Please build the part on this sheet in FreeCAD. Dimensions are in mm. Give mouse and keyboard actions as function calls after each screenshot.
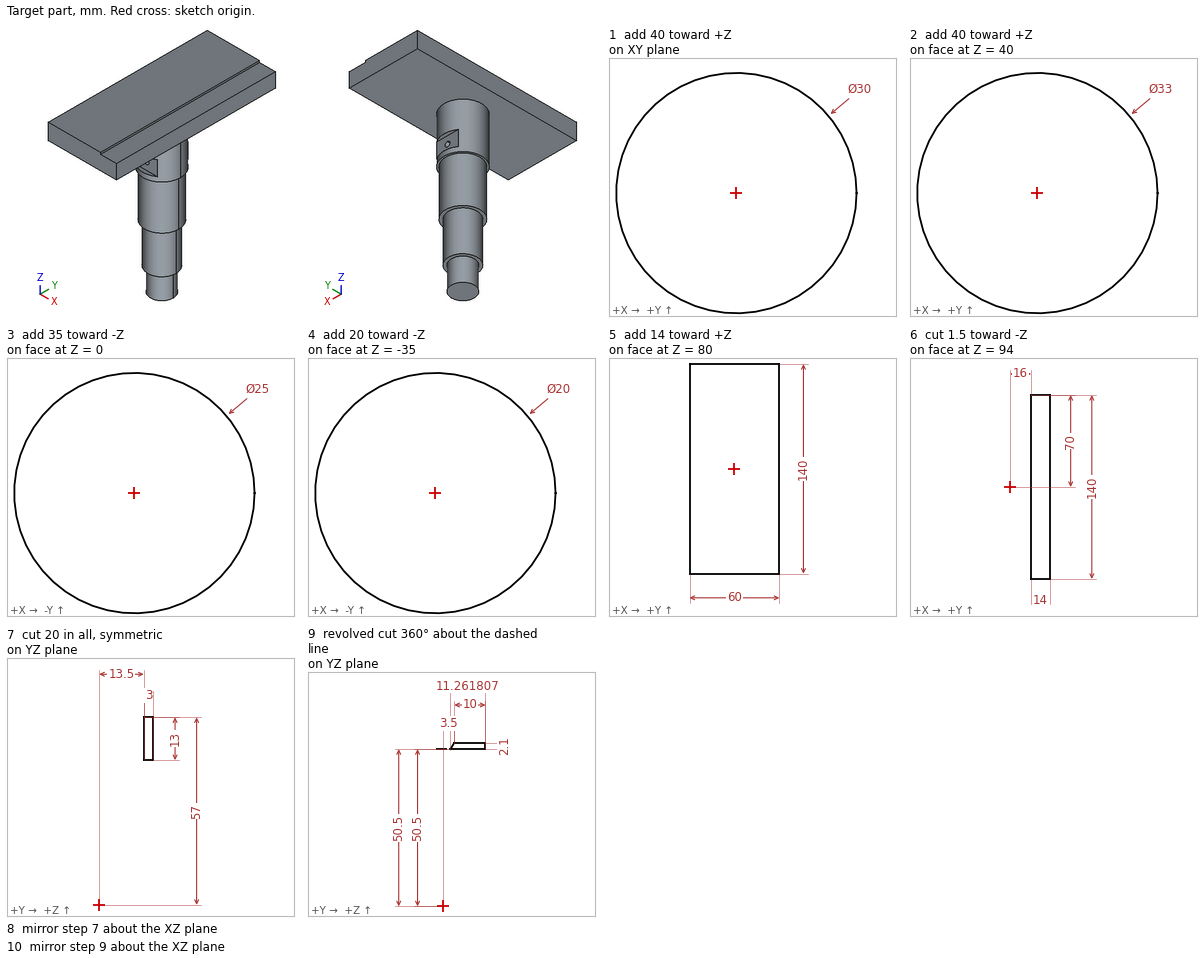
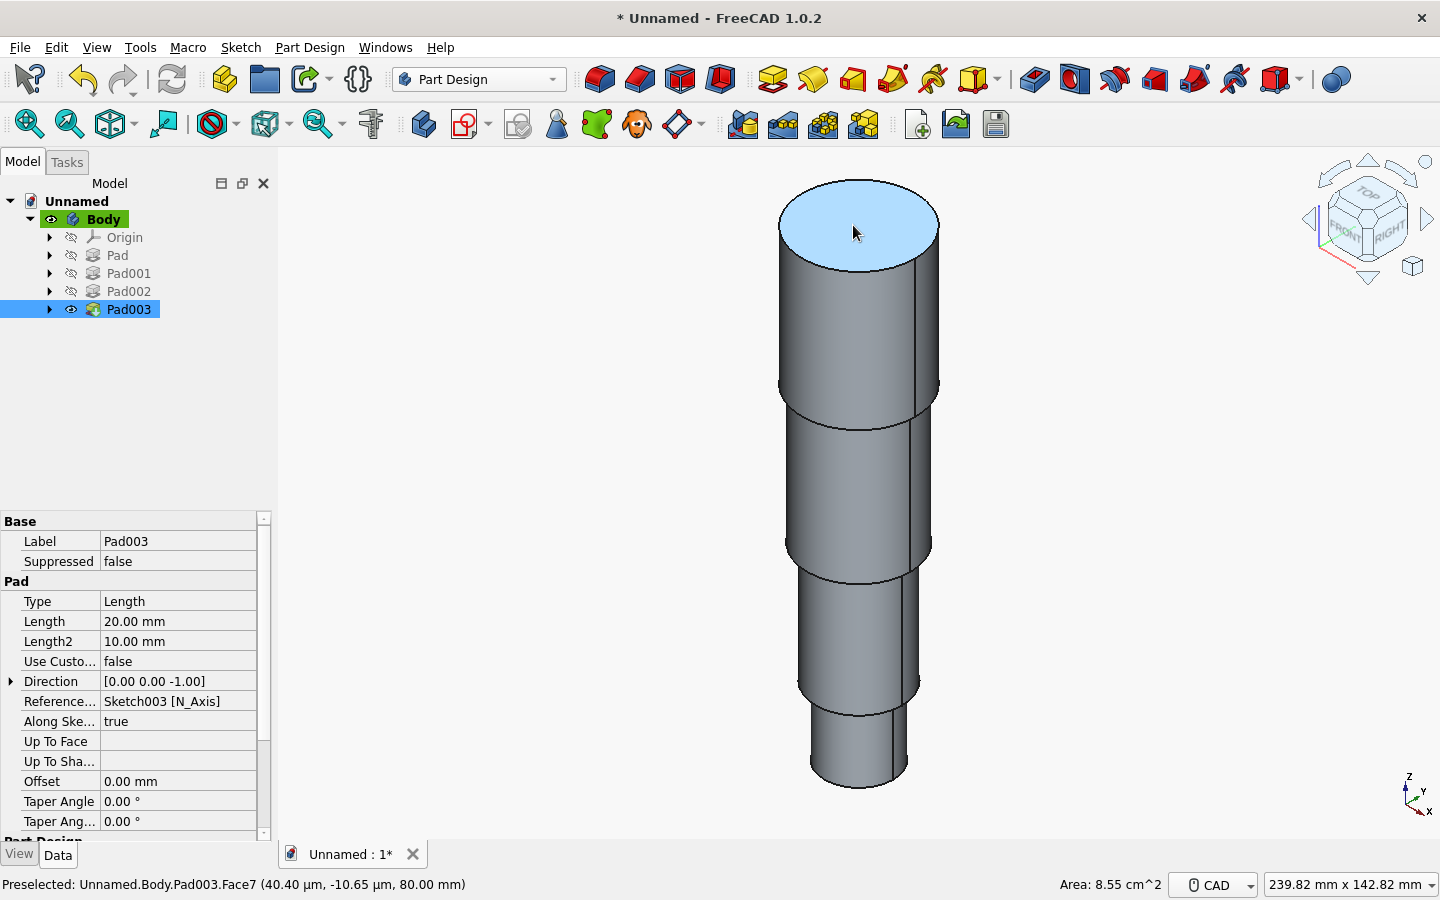
click(464, 124)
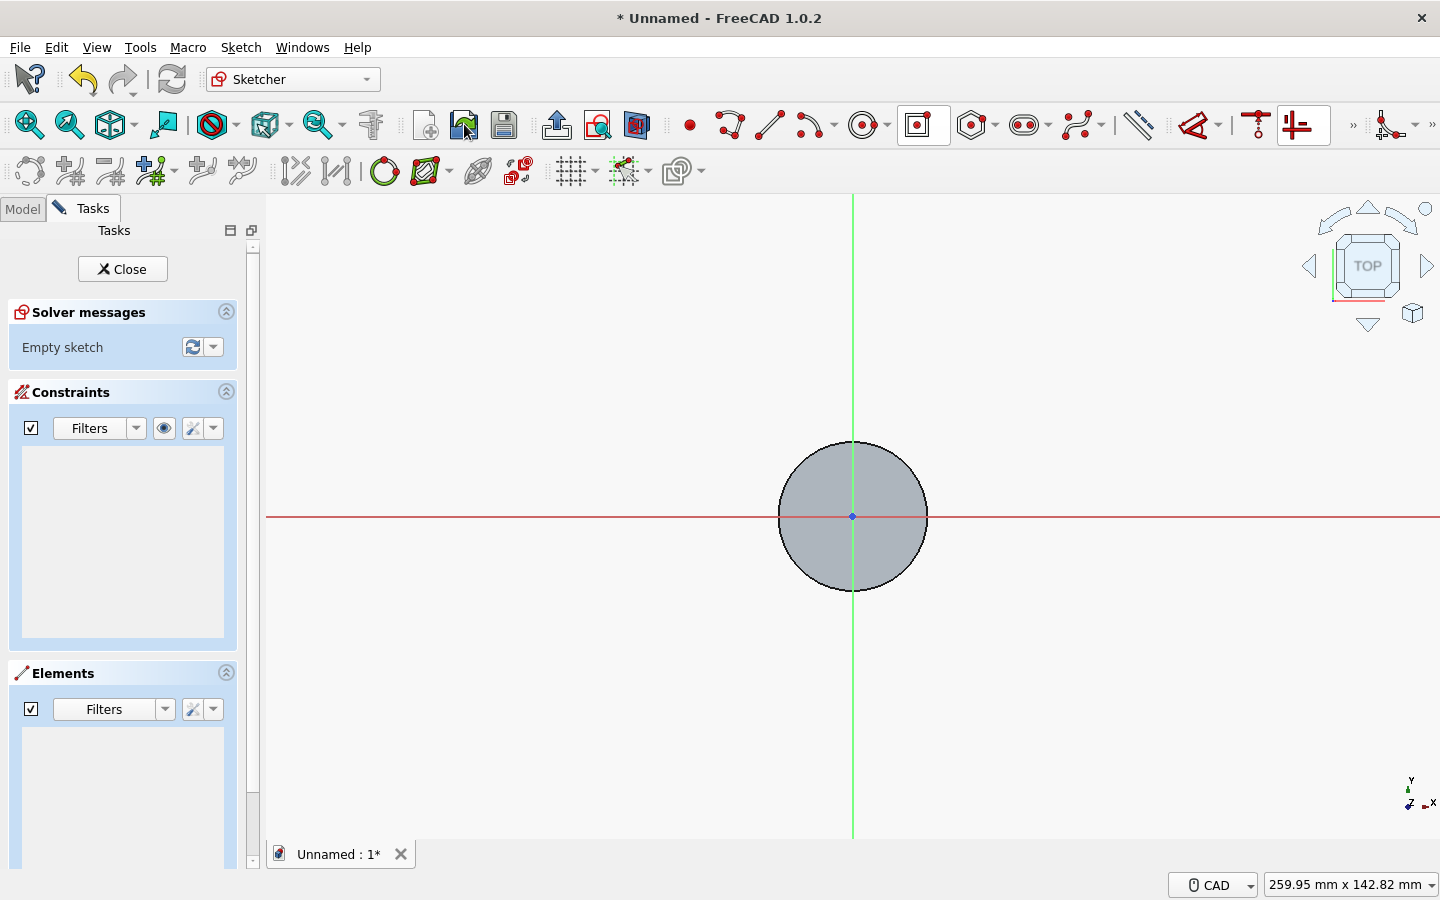
scroll(645, 516, down, 2)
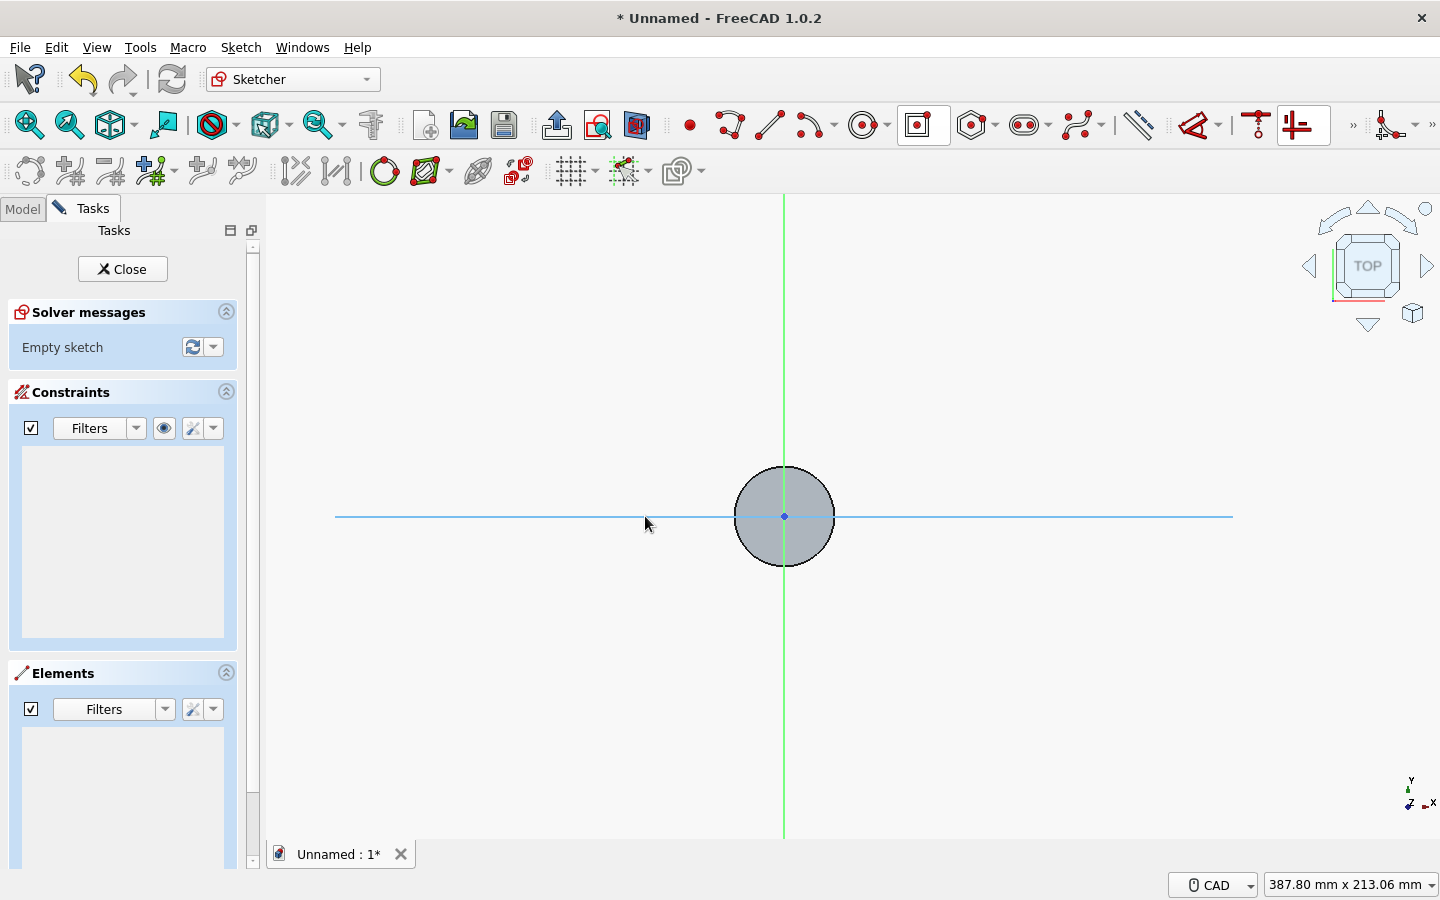
click(918, 126)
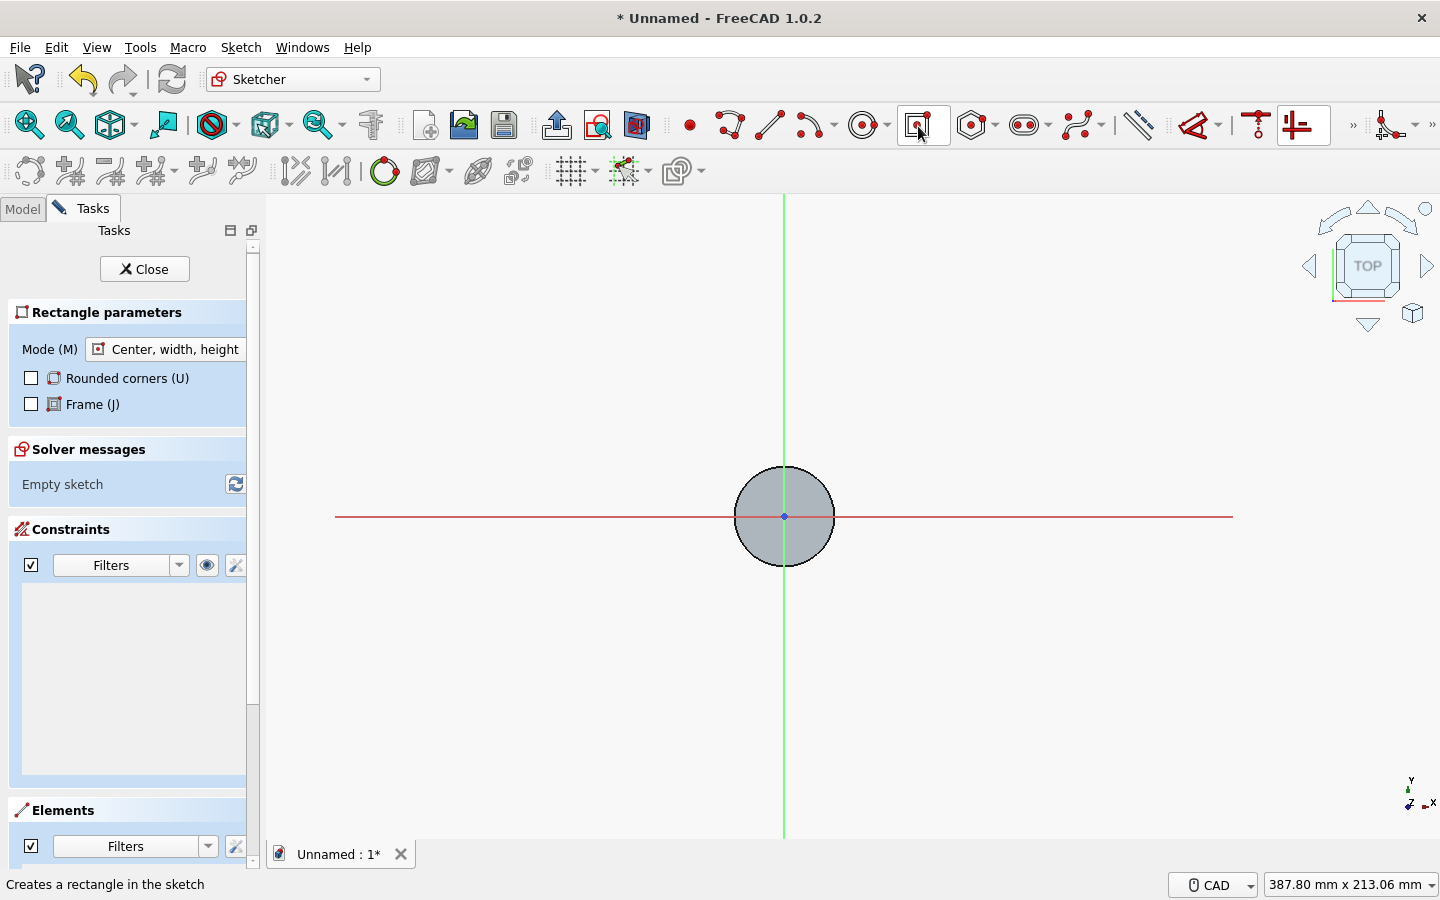
click(784, 516)
move(875, 305)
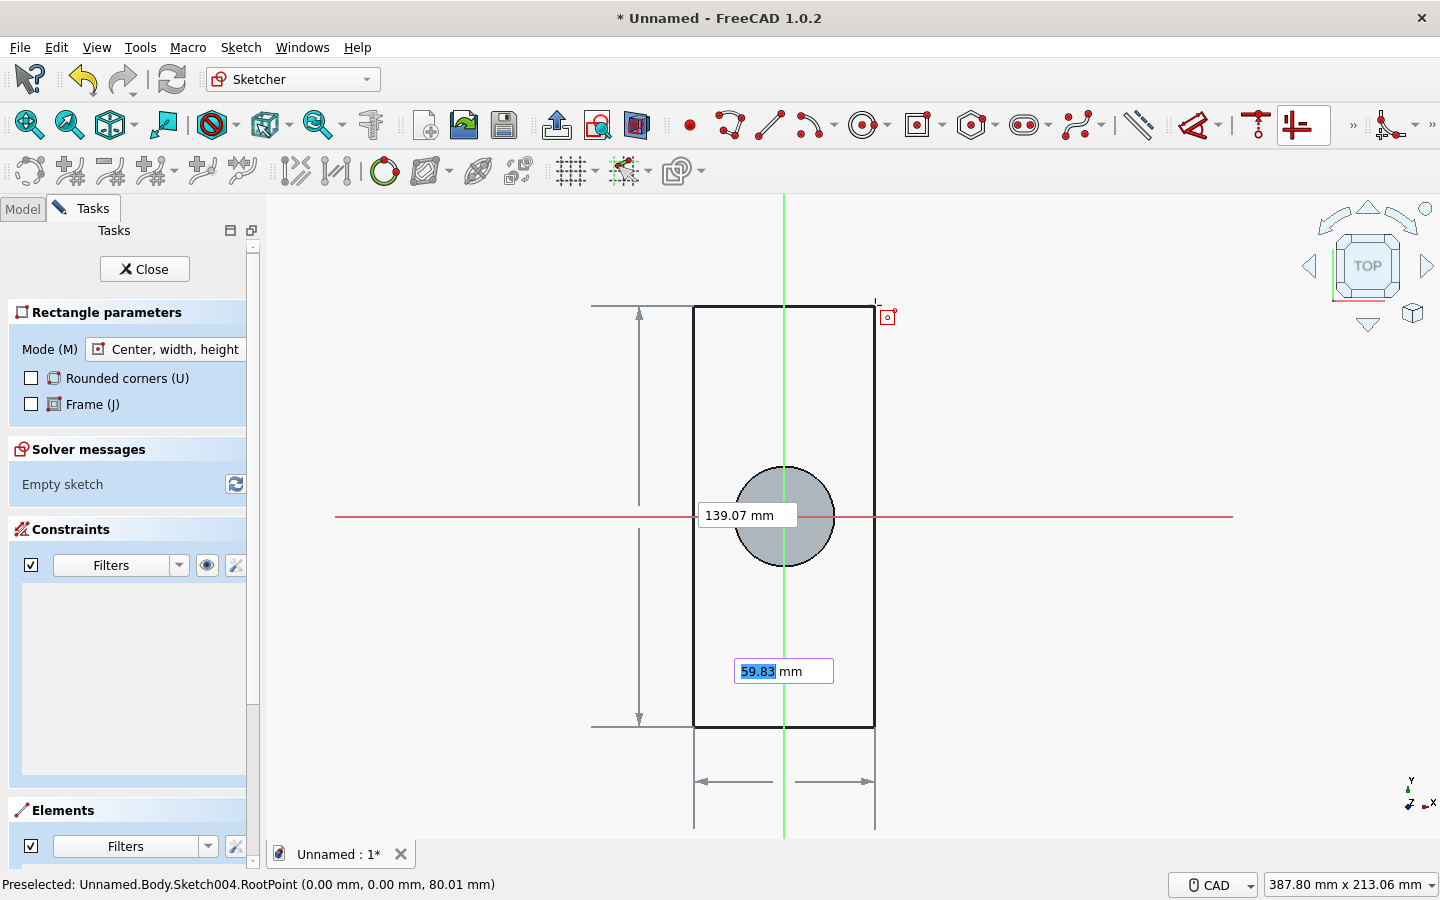
text(60)
key(Tab)
text(140)
key(Return)
key(Escape)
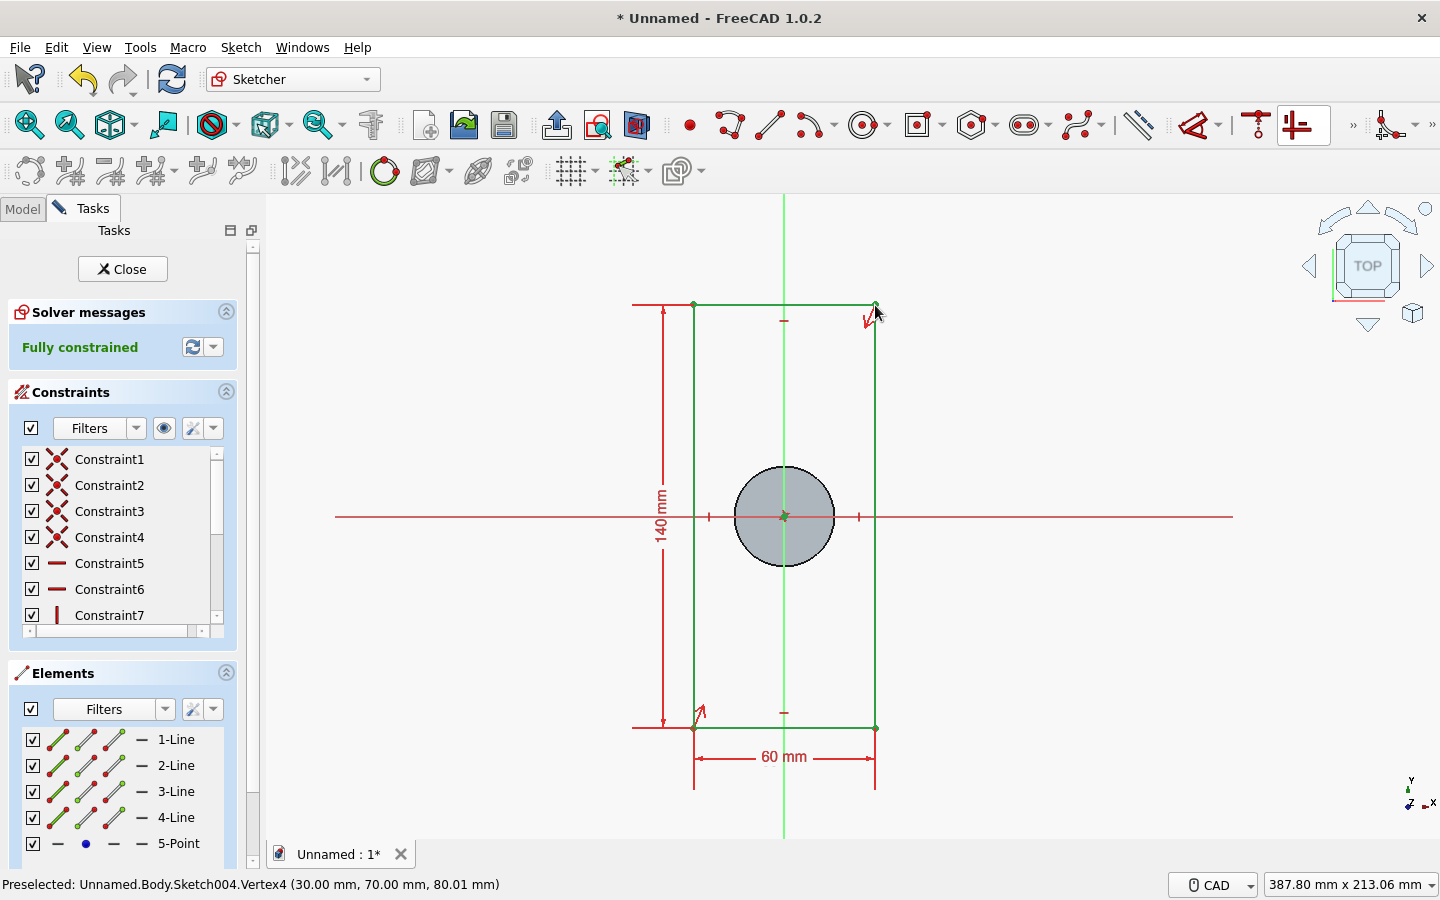
click(123, 269)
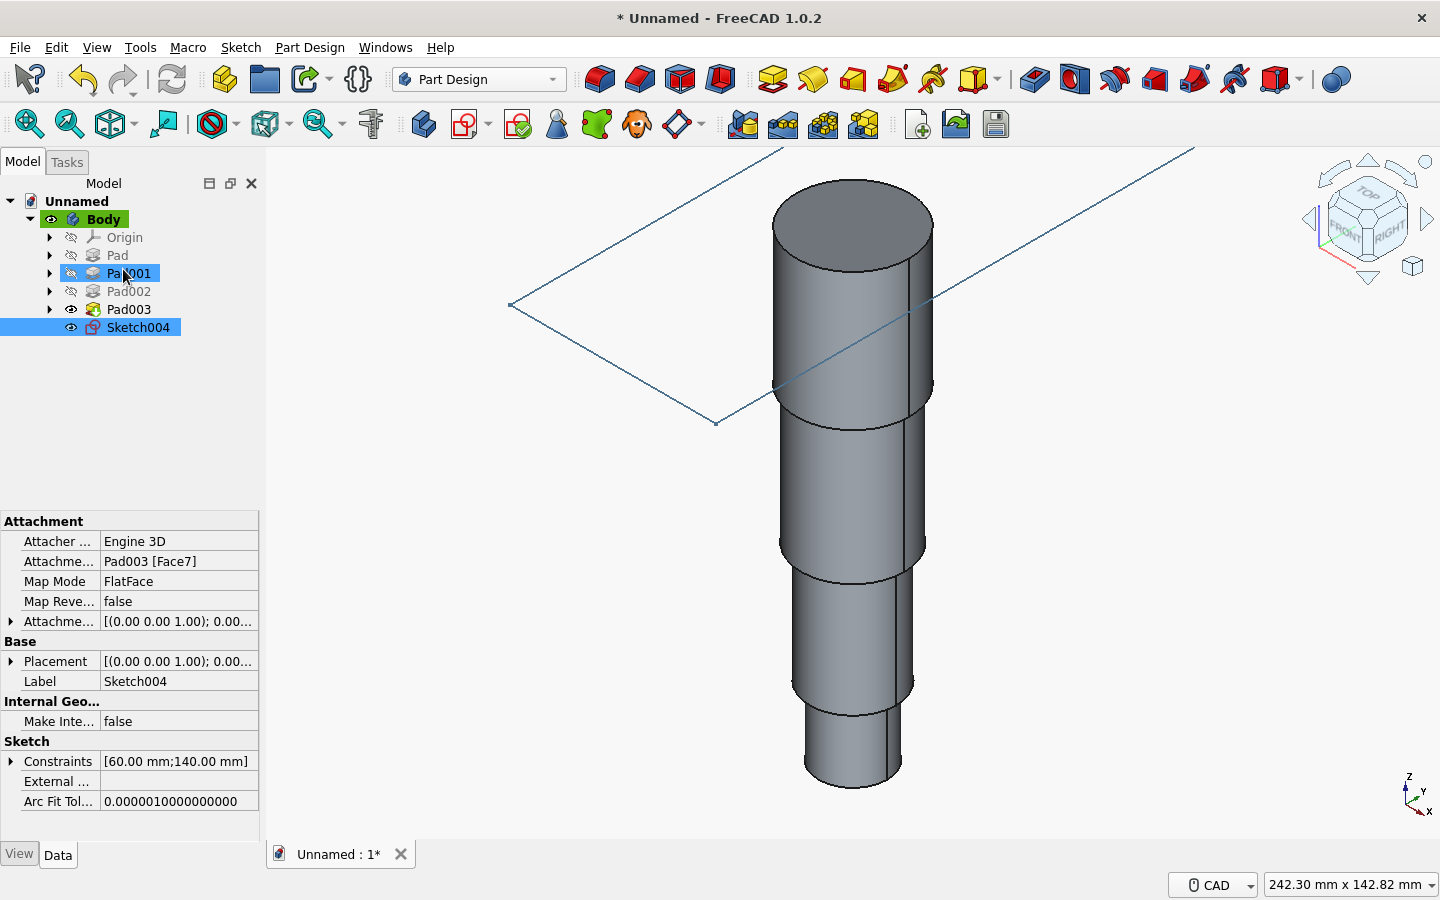
click(774, 80)